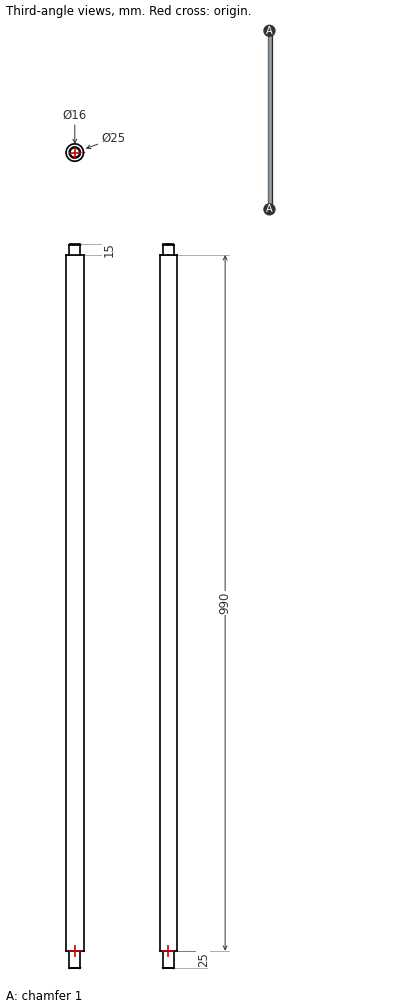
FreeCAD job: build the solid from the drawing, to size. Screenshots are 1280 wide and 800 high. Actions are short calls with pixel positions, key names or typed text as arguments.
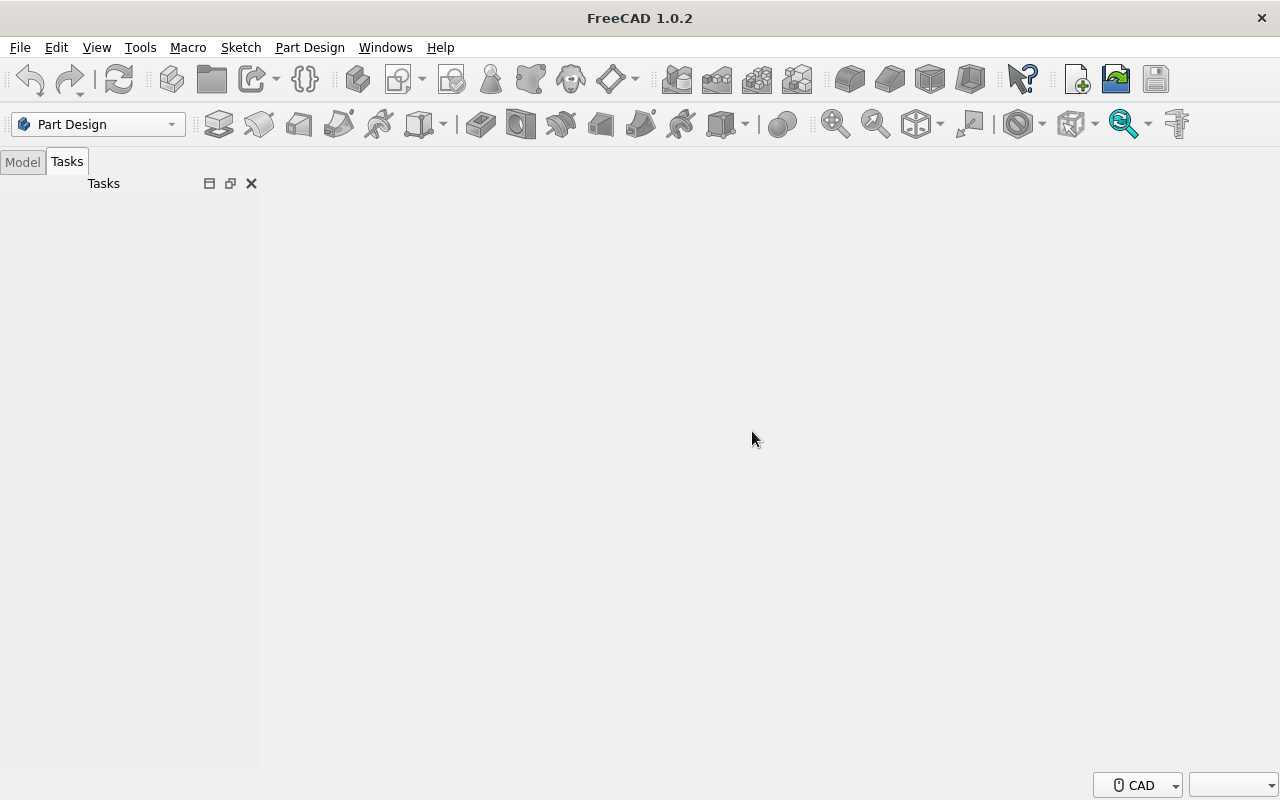
click(1076, 80)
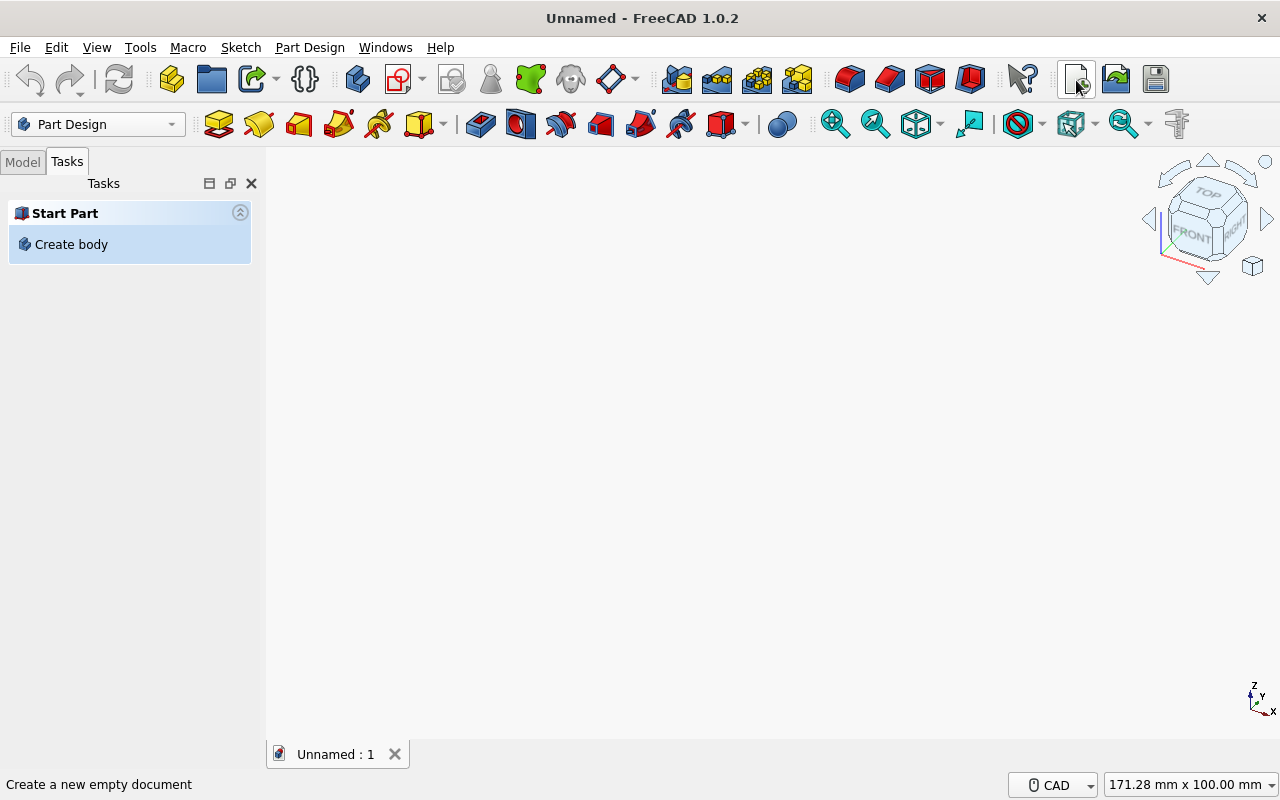
click(398, 80)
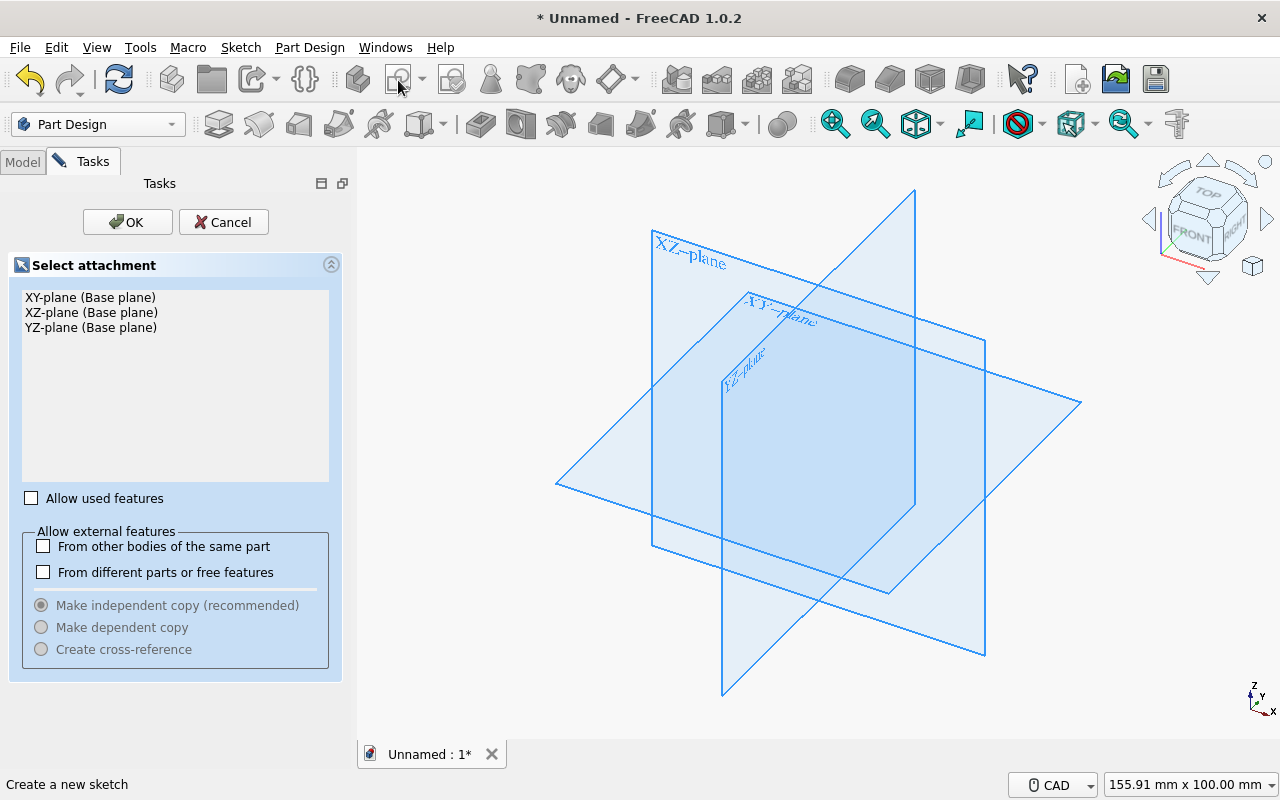
click(82, 298)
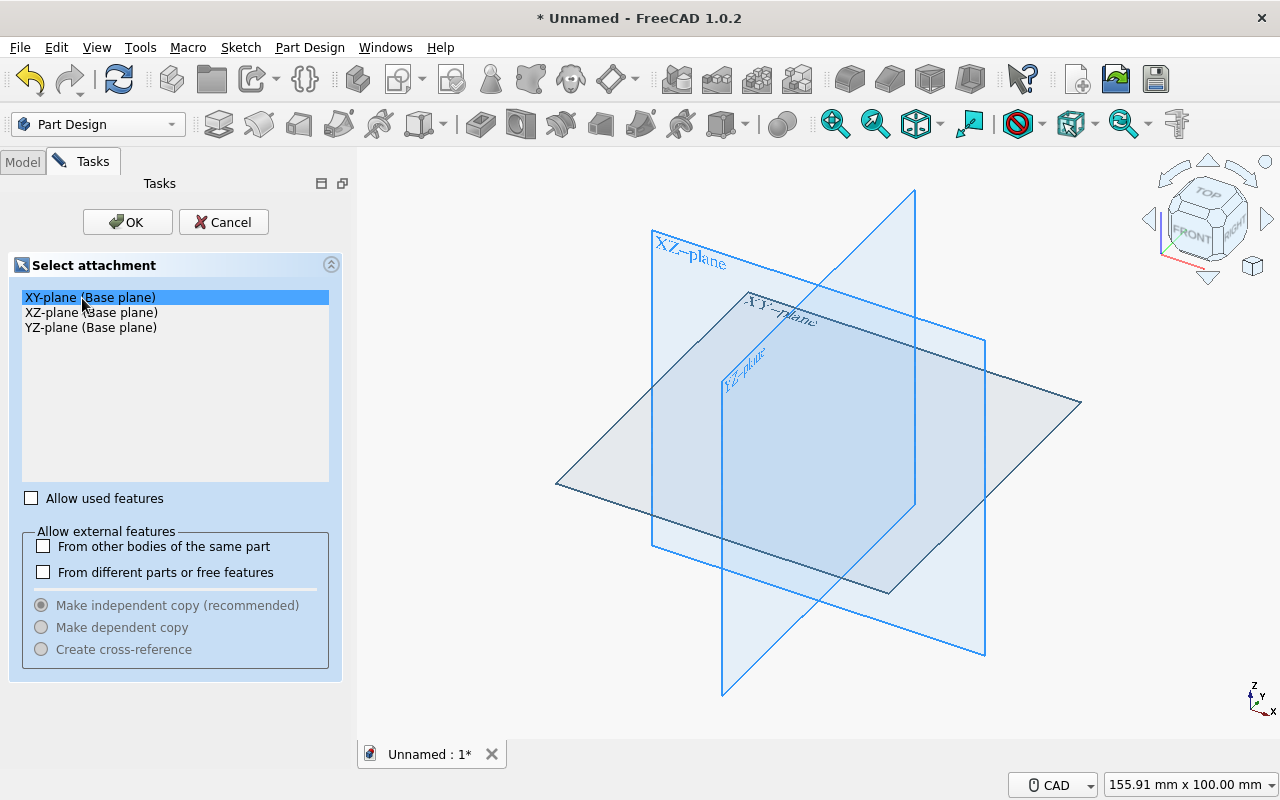
click(128, 222)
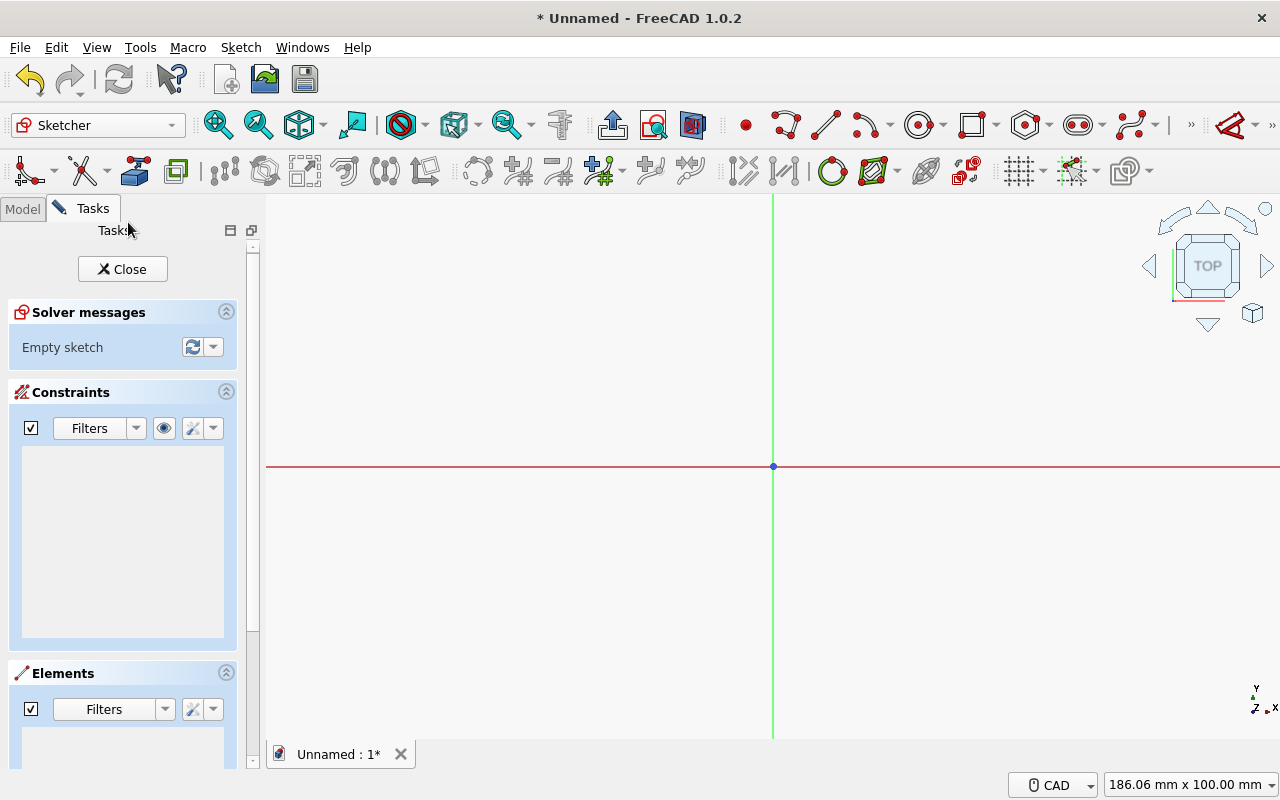
scroll(813, 466, up, 5)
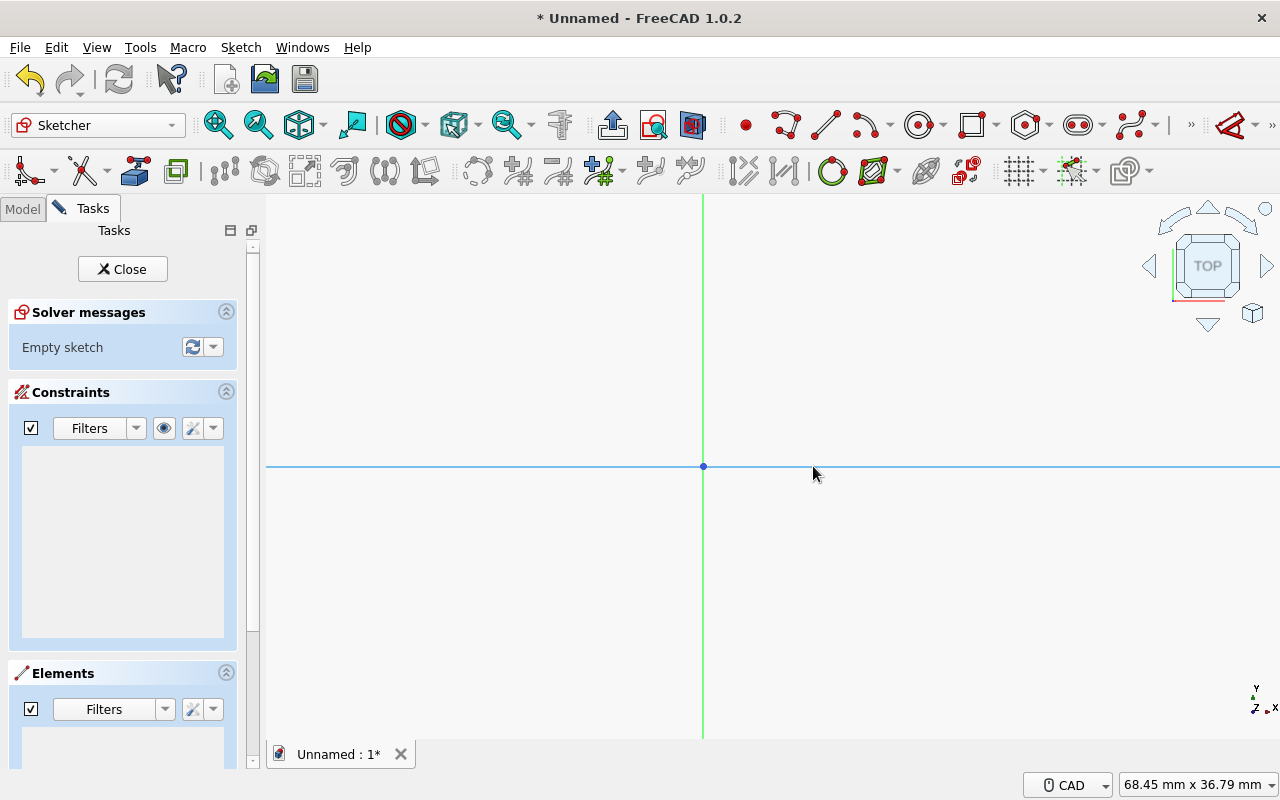
click(920, 126)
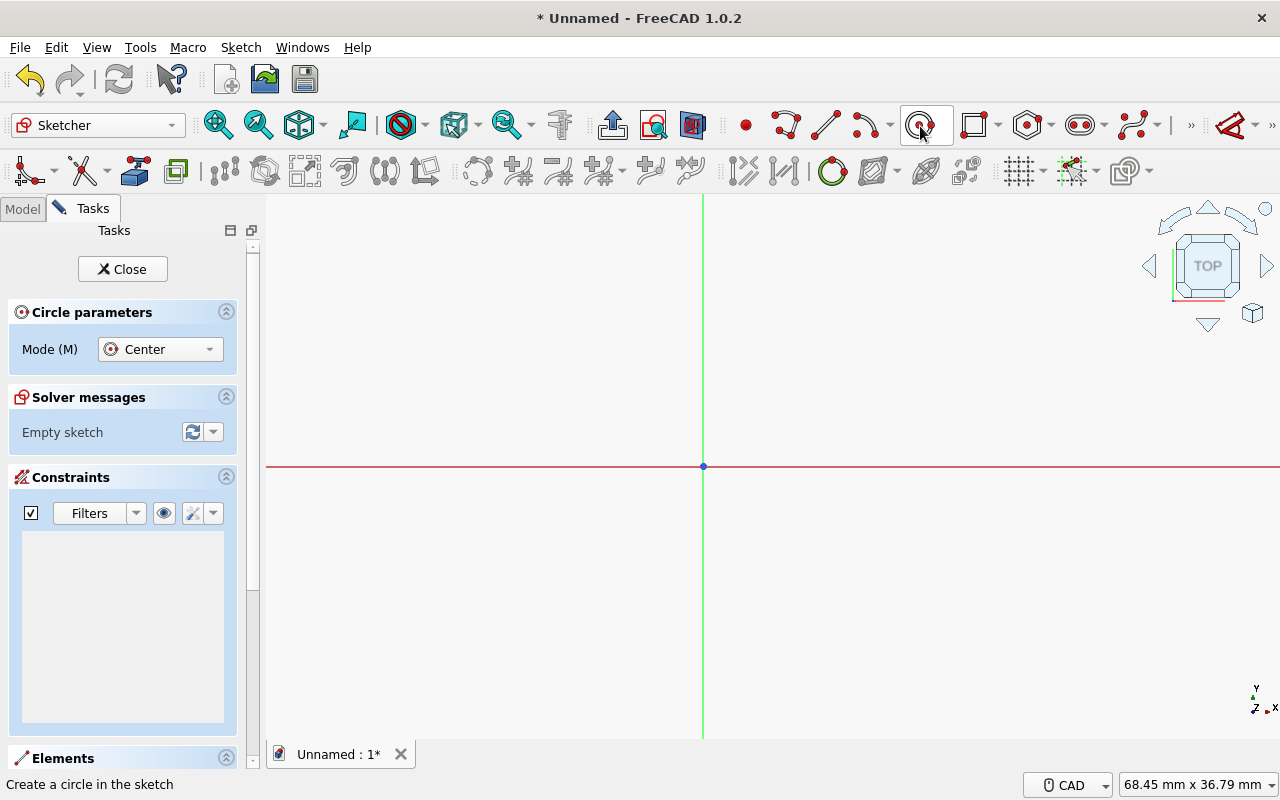
click(703, 466)
move(834, 336)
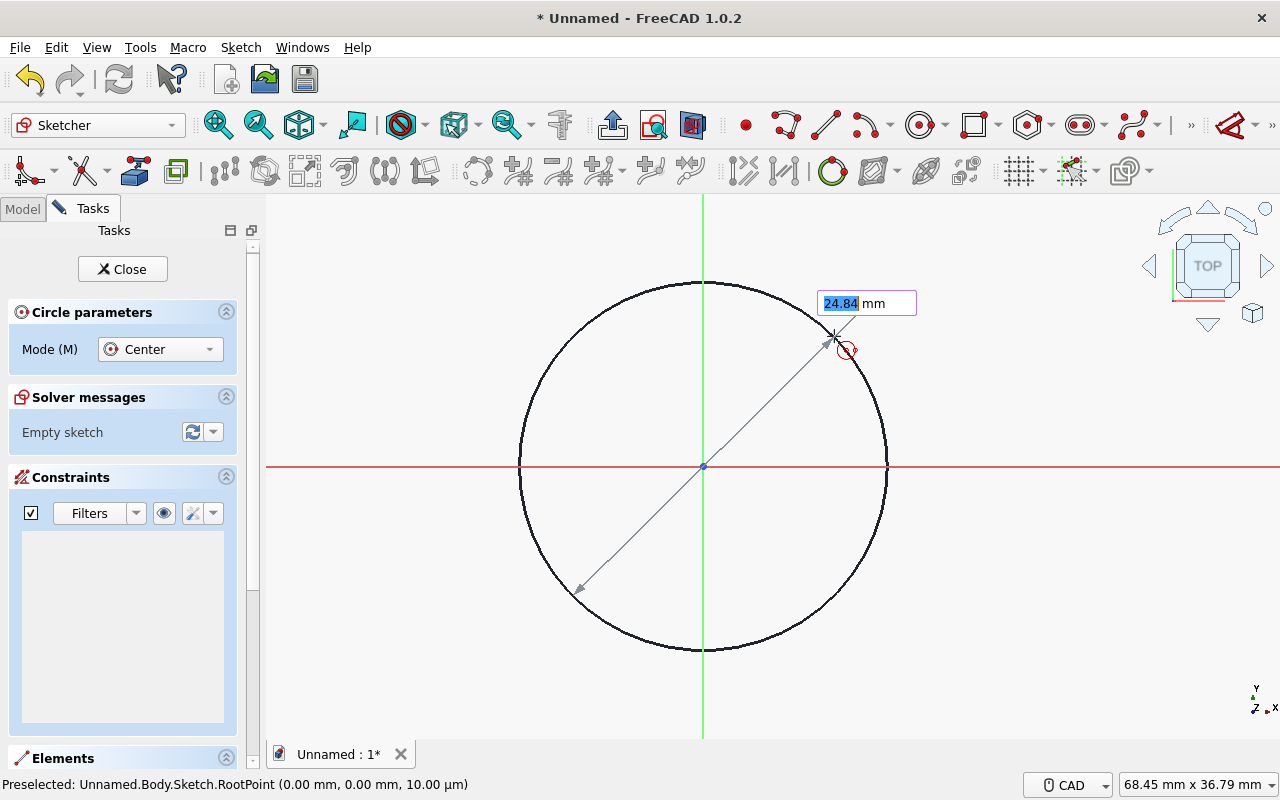
text(25)
key(Return)
key(Escape)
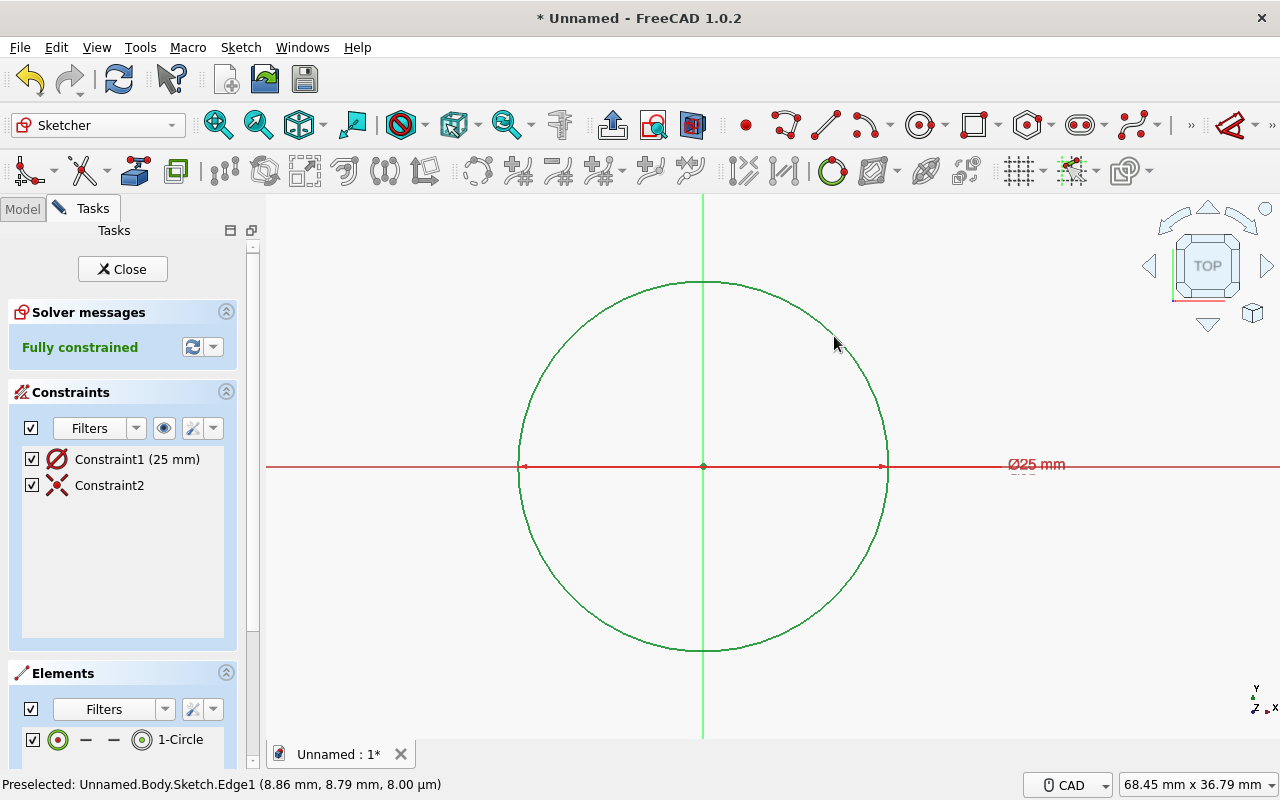
click(123, 269)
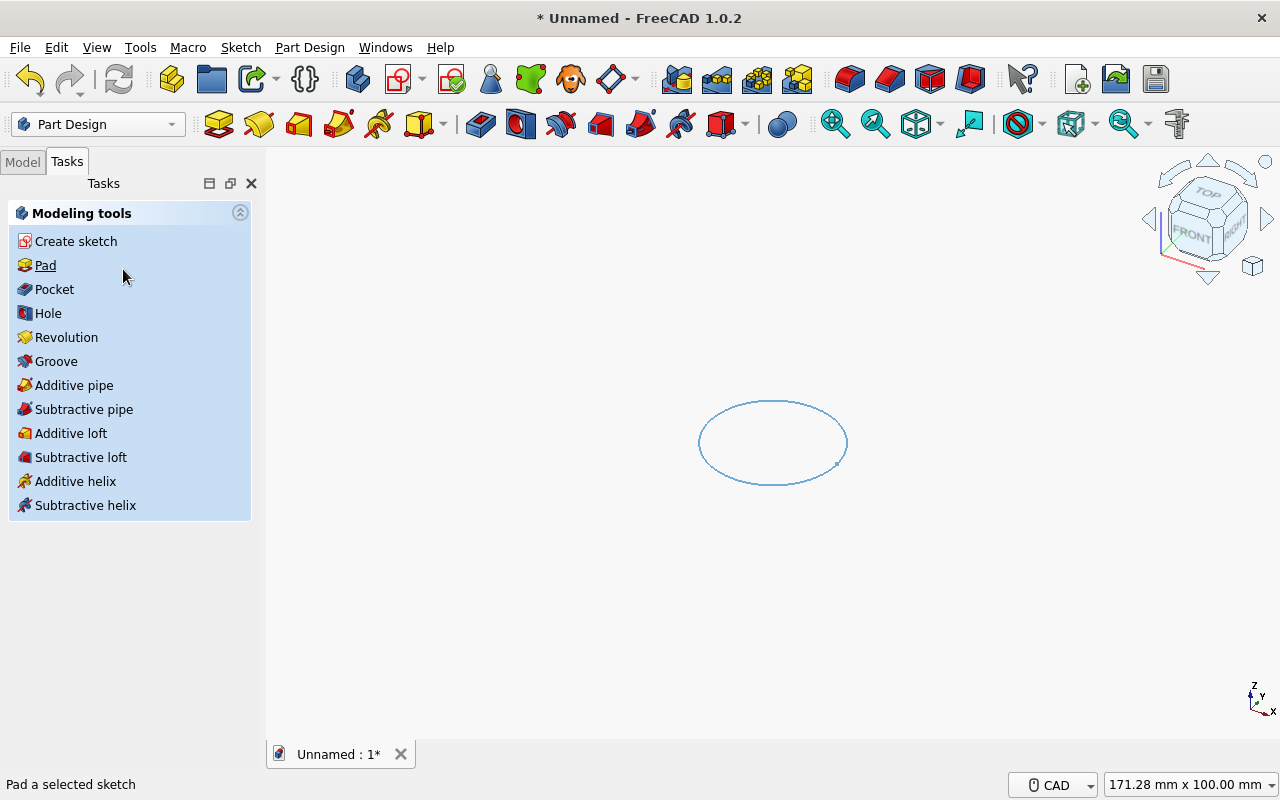
click(220, 124)